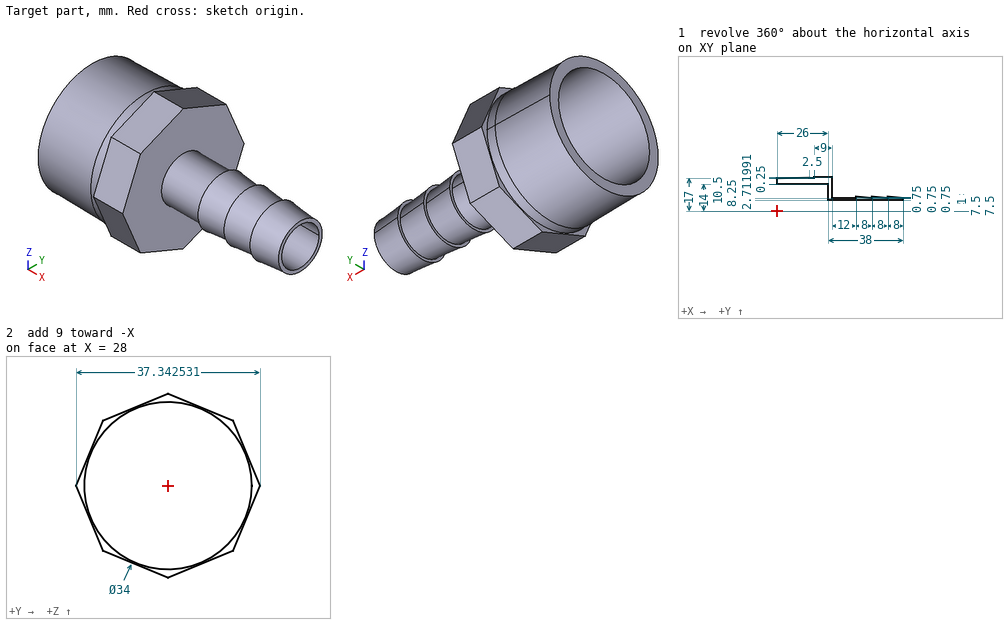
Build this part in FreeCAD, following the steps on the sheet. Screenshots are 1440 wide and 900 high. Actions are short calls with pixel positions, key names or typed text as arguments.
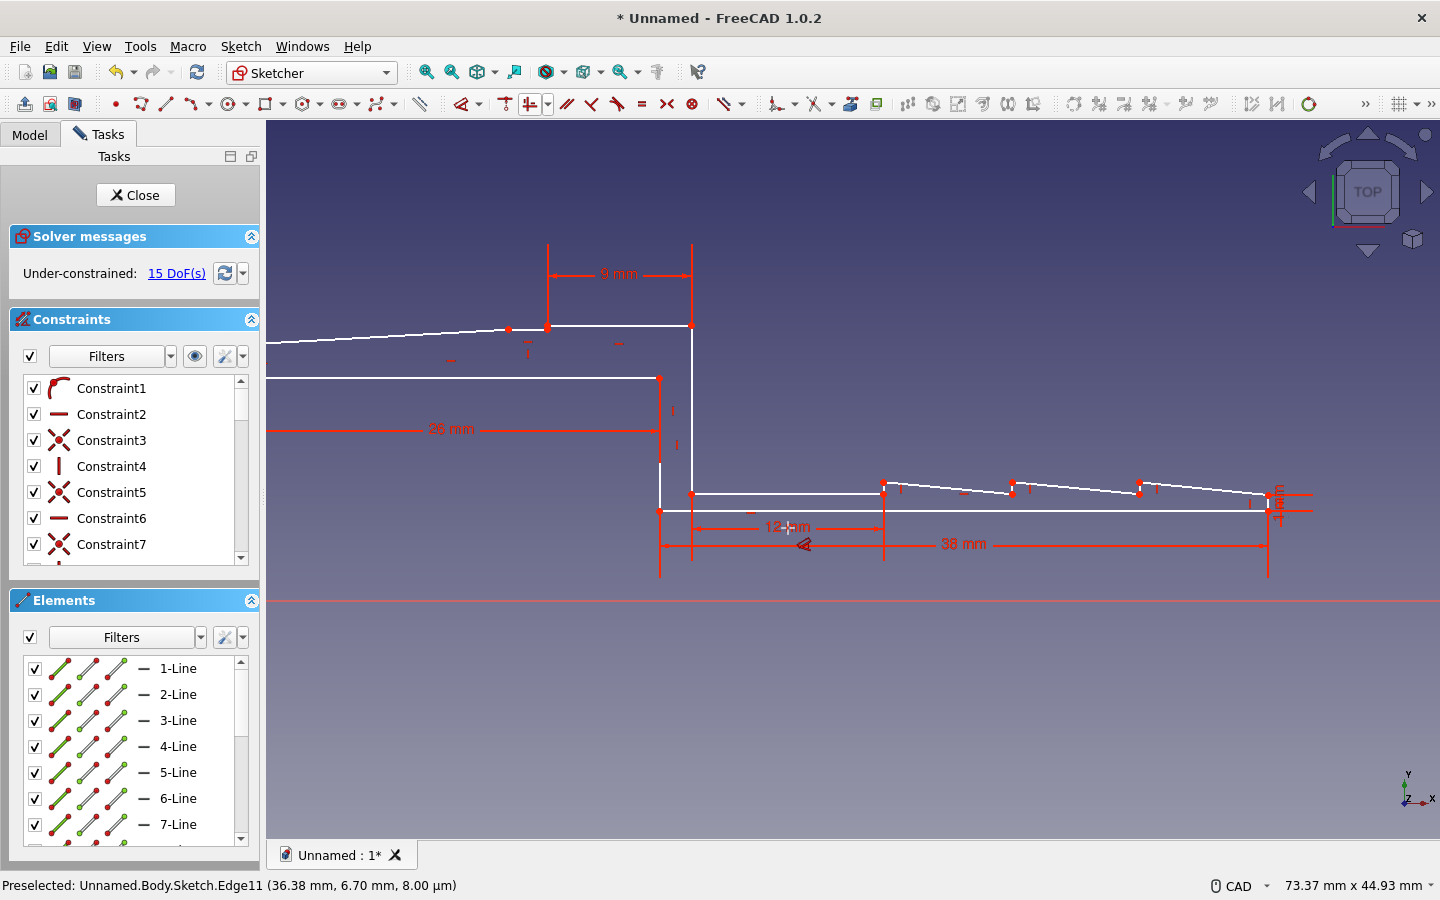
click(1230, 491)
click(1204, 529)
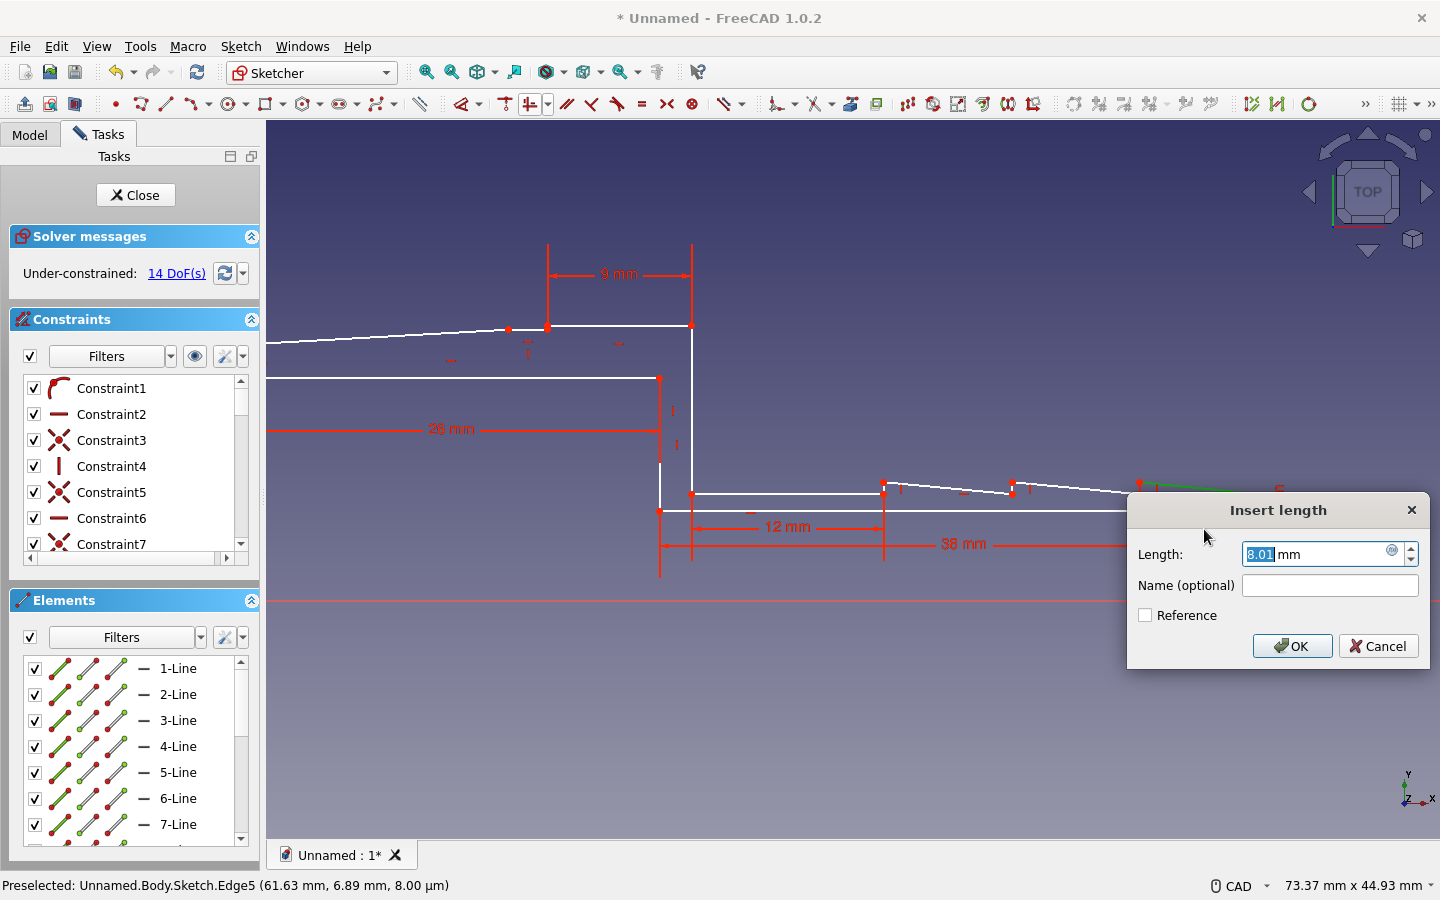
text(8)
key(Return)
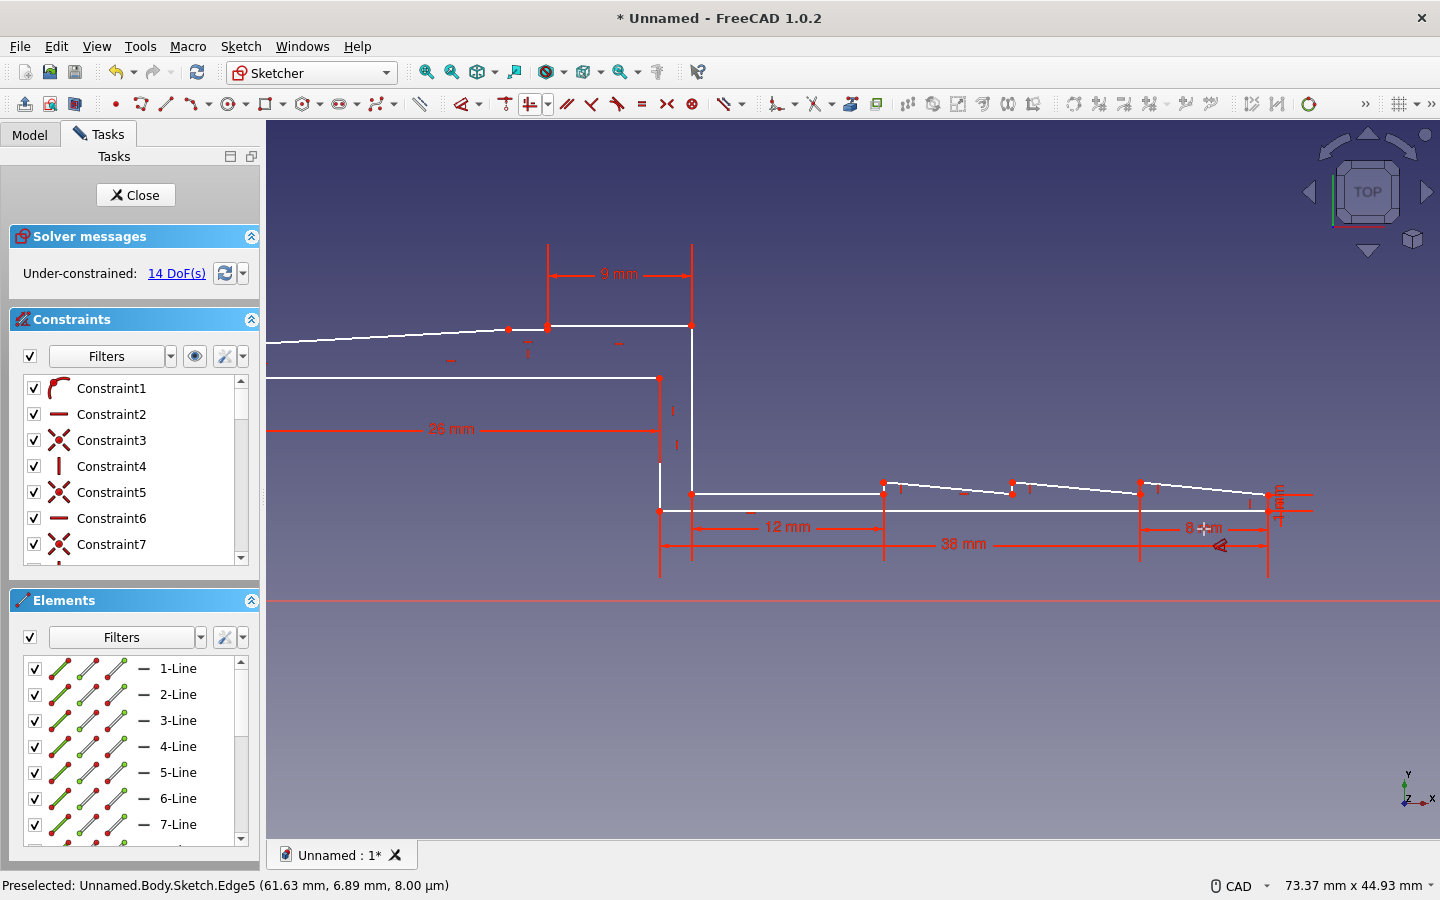
click(1102, 491)
click(1076, 528)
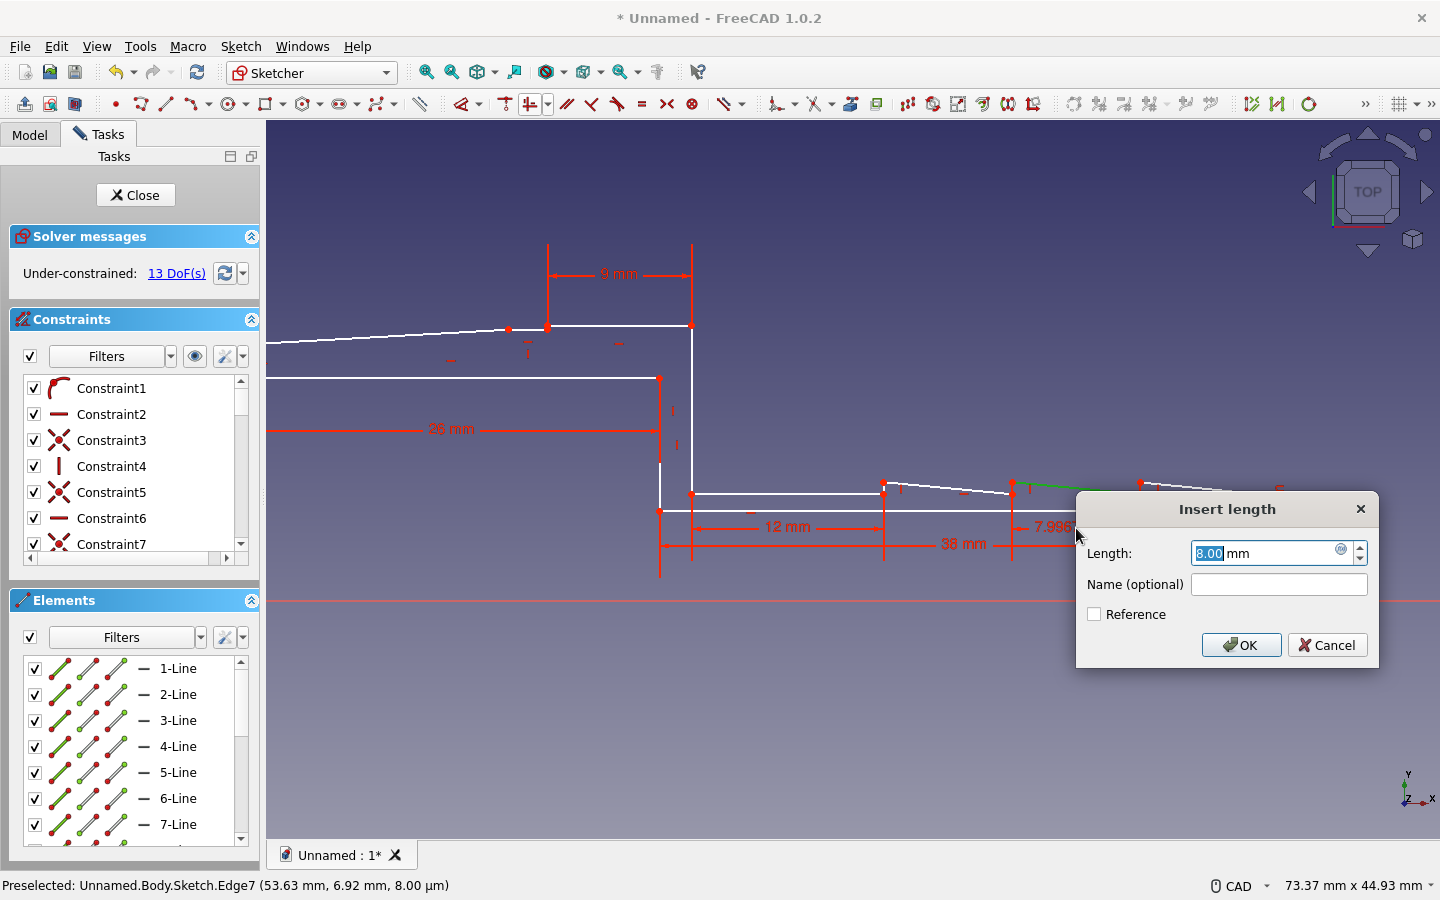
text(8)
key(Return)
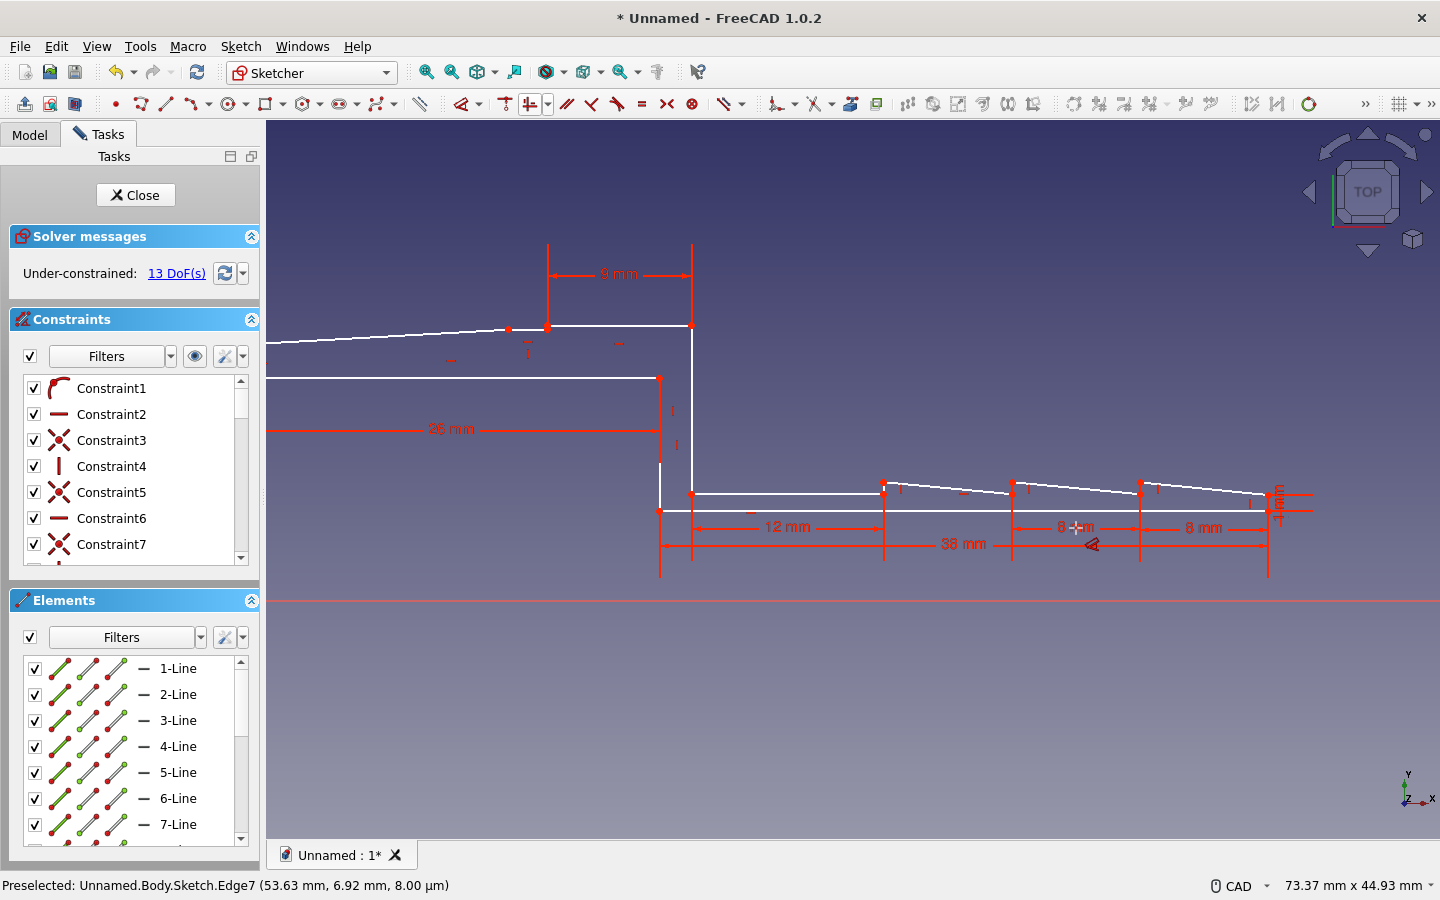
click(974, 491)
click(948, 448)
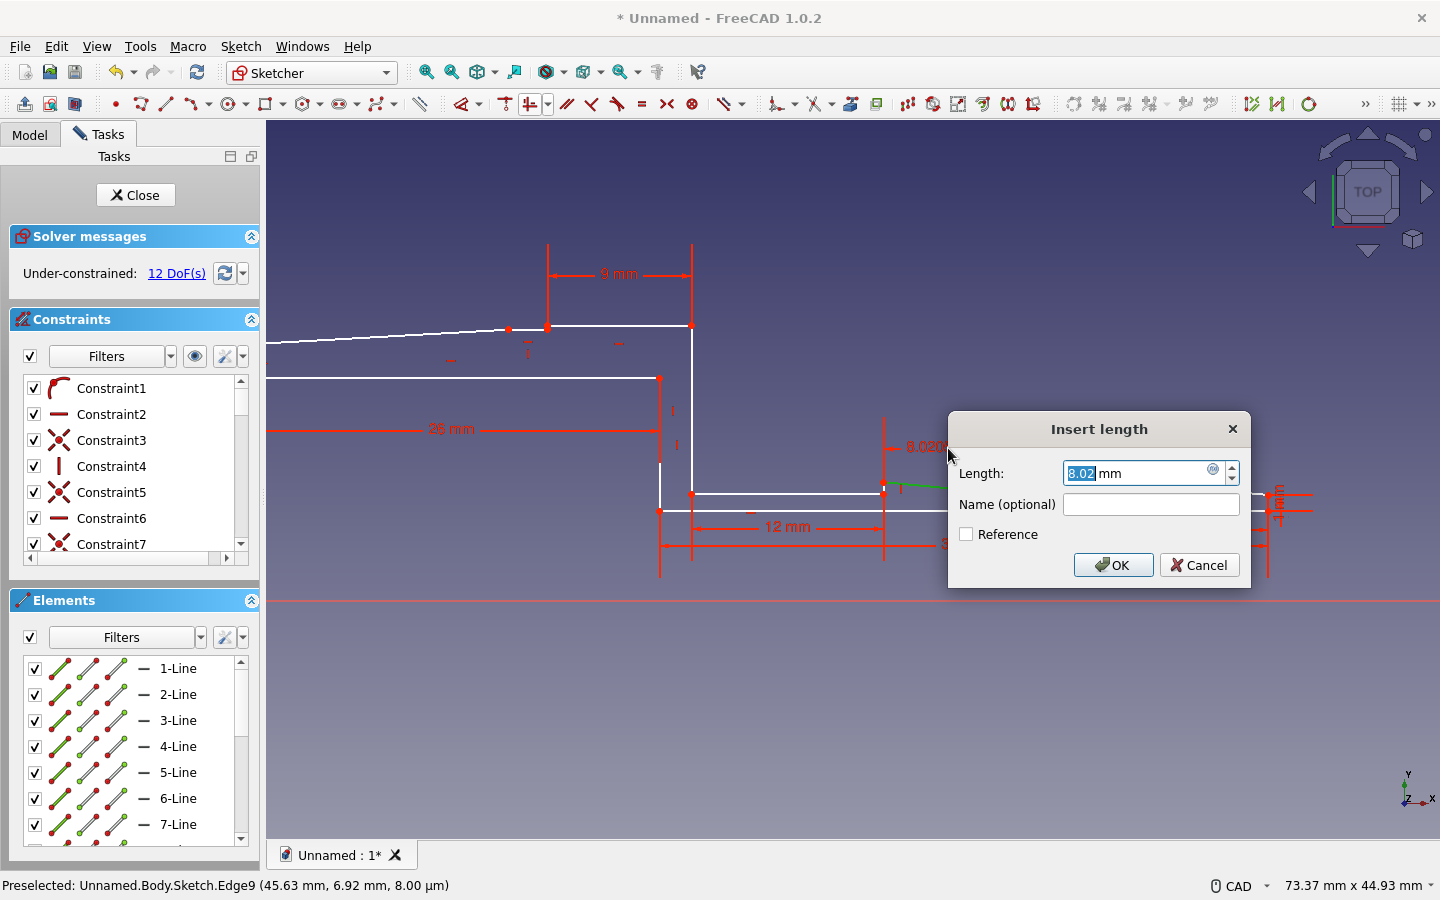
text(8)
key(Return)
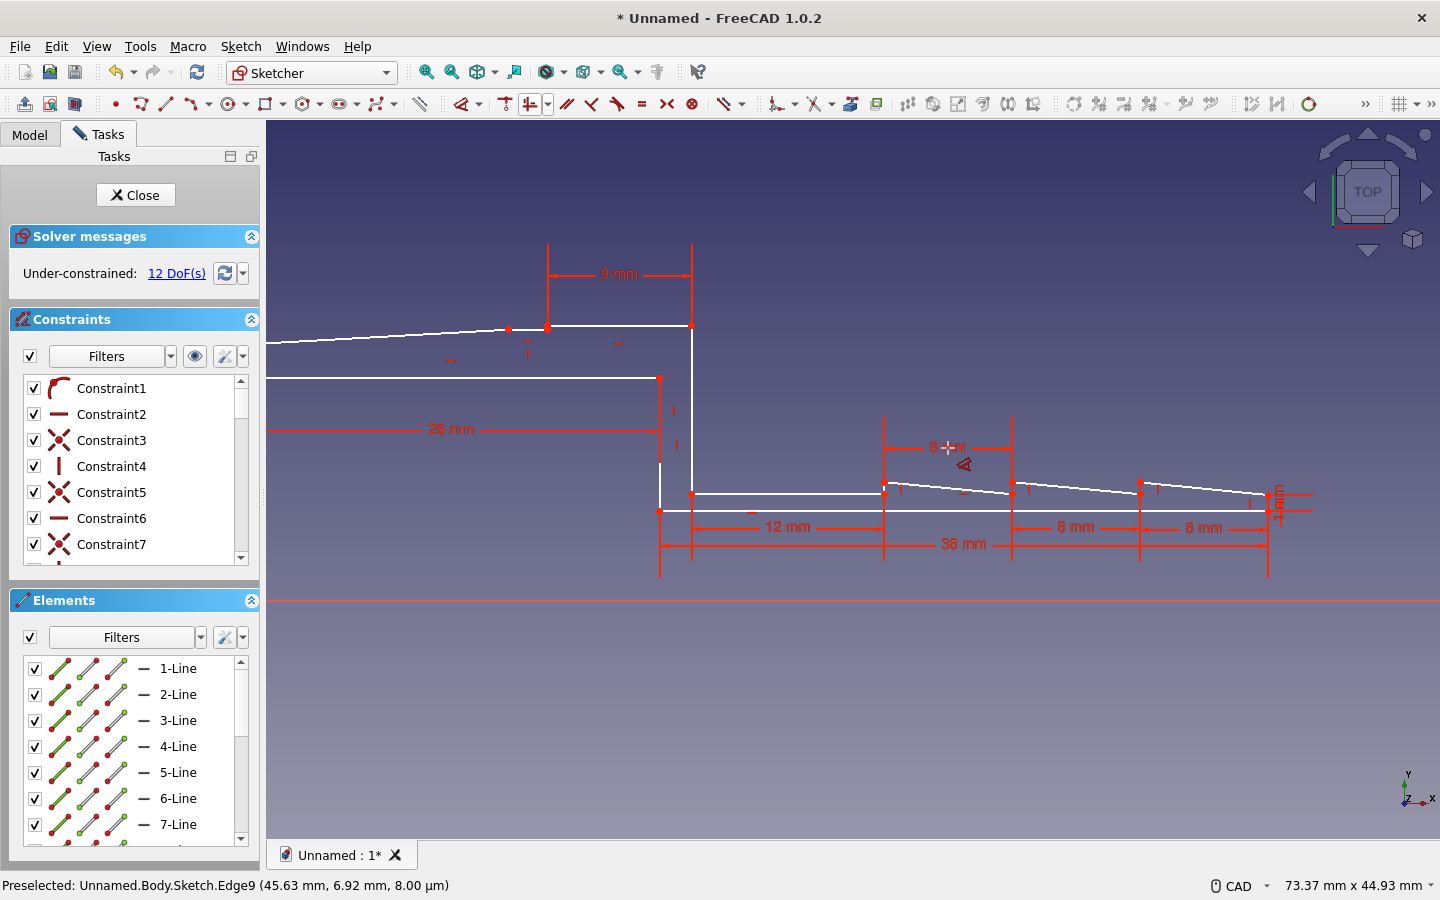
click(536, 330)
click(528, 296)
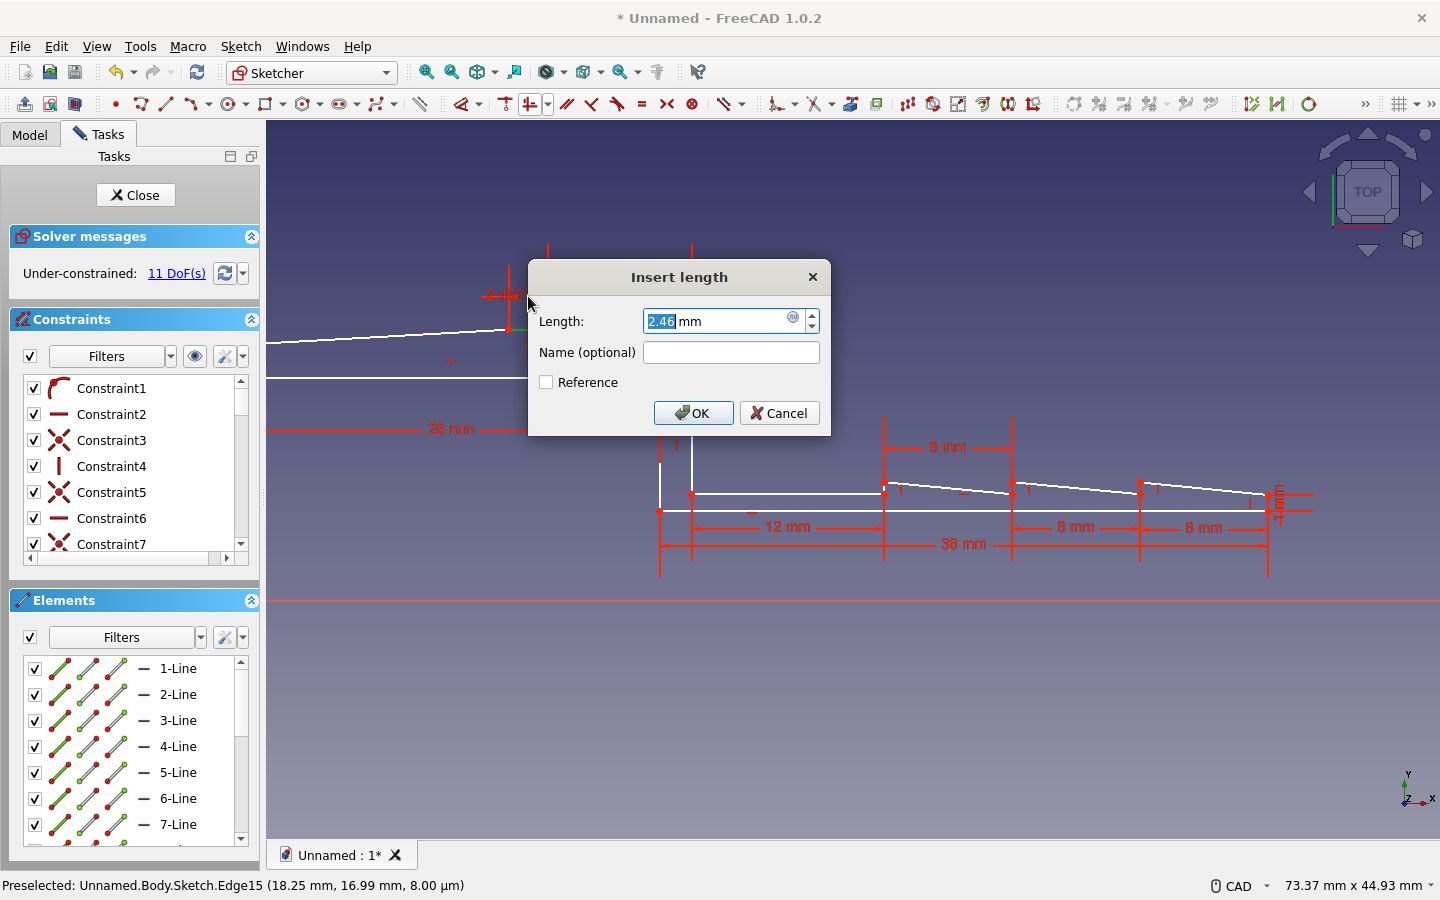
text(2.5)
key(Return)